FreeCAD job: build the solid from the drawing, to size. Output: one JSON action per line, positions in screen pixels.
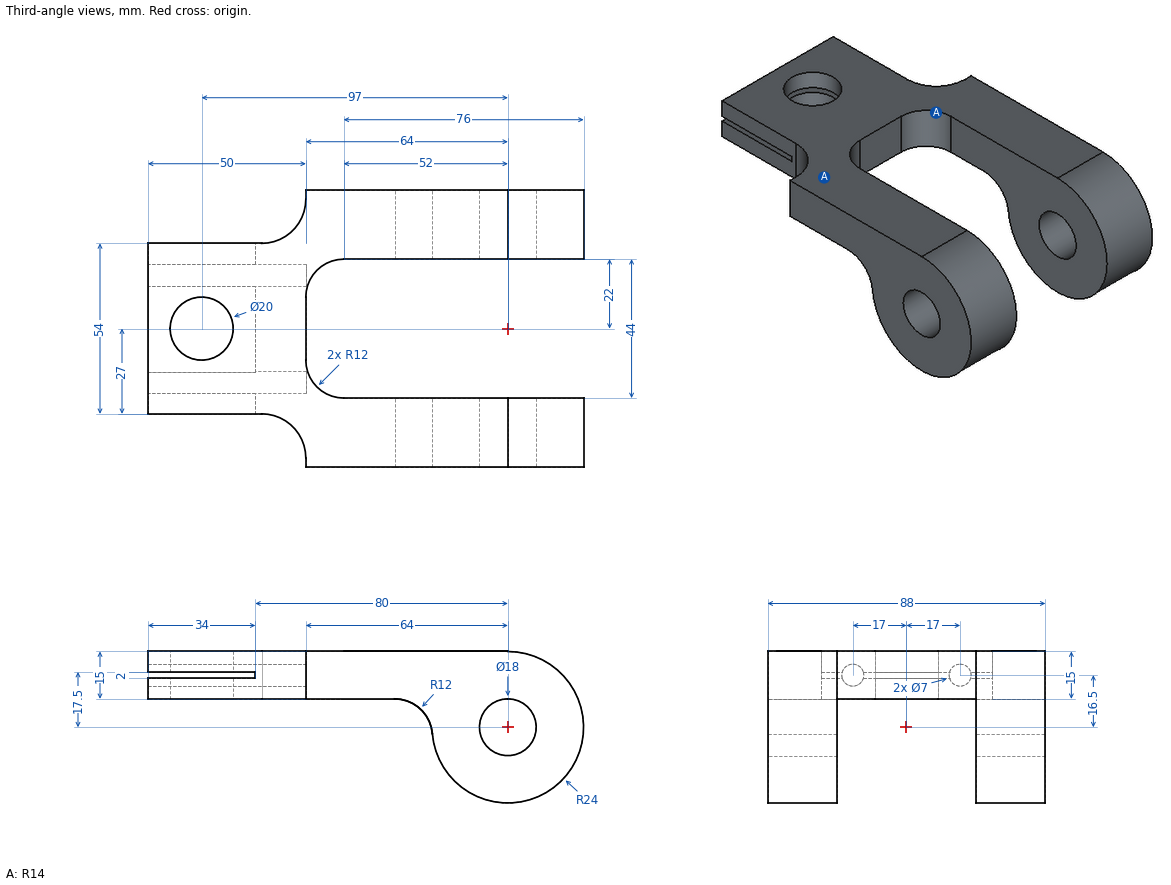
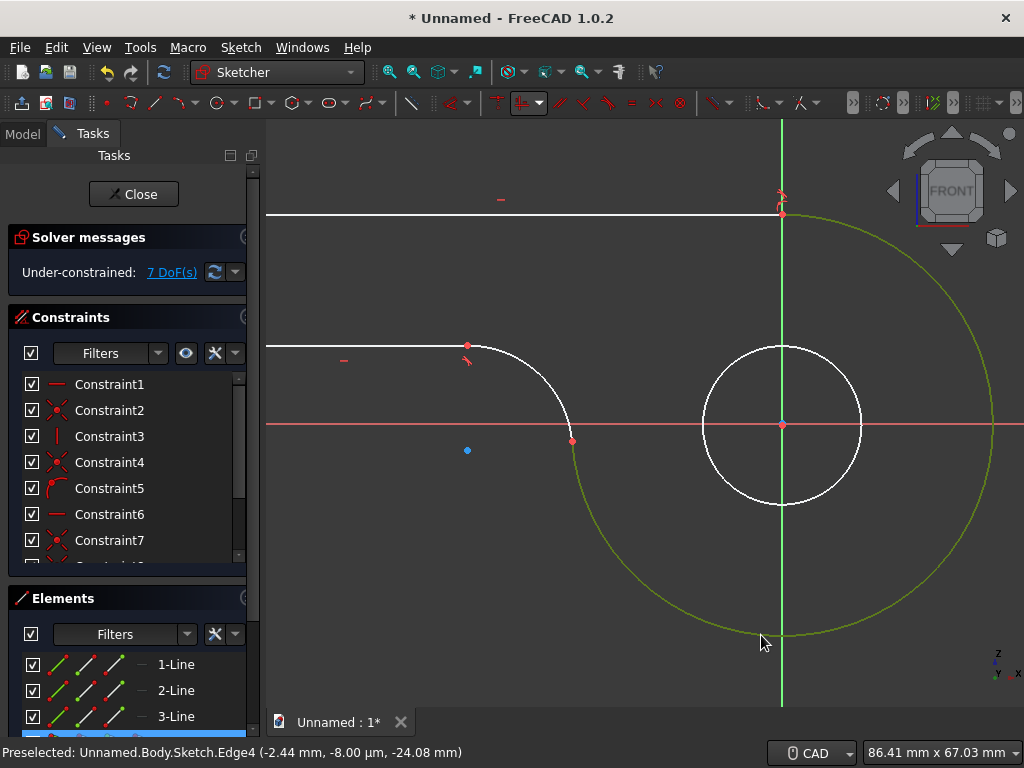
{"action": "left_click", "coordinate": [558, 398]}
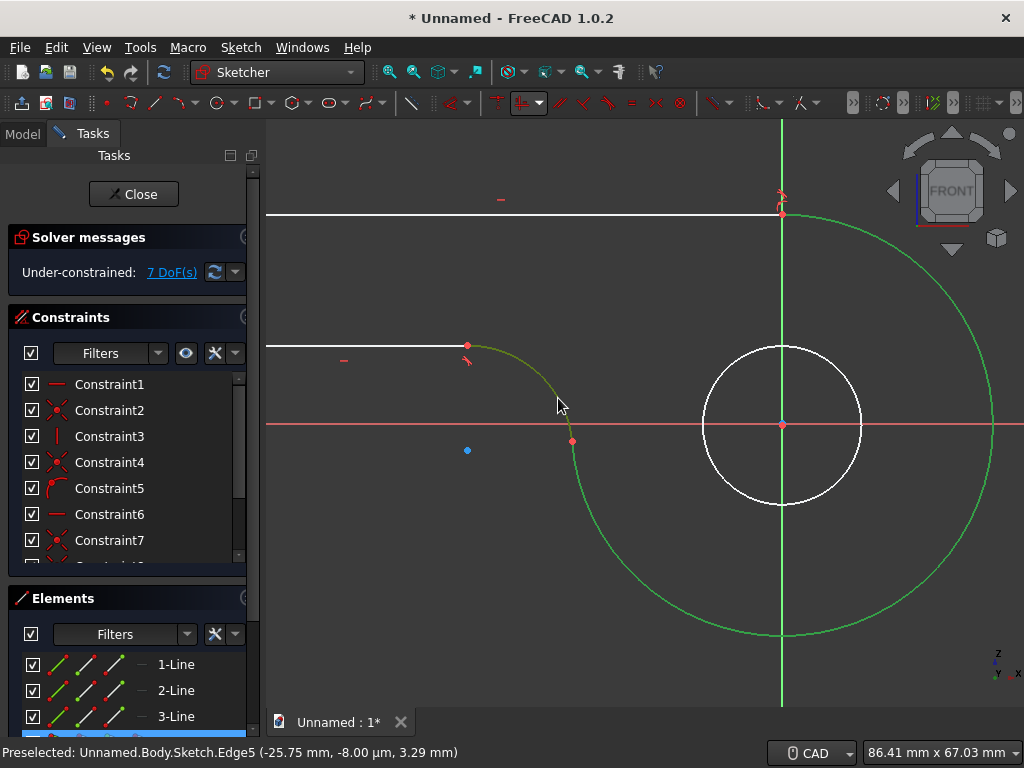
{"action": "left_click", "coordinate": [608, 104]}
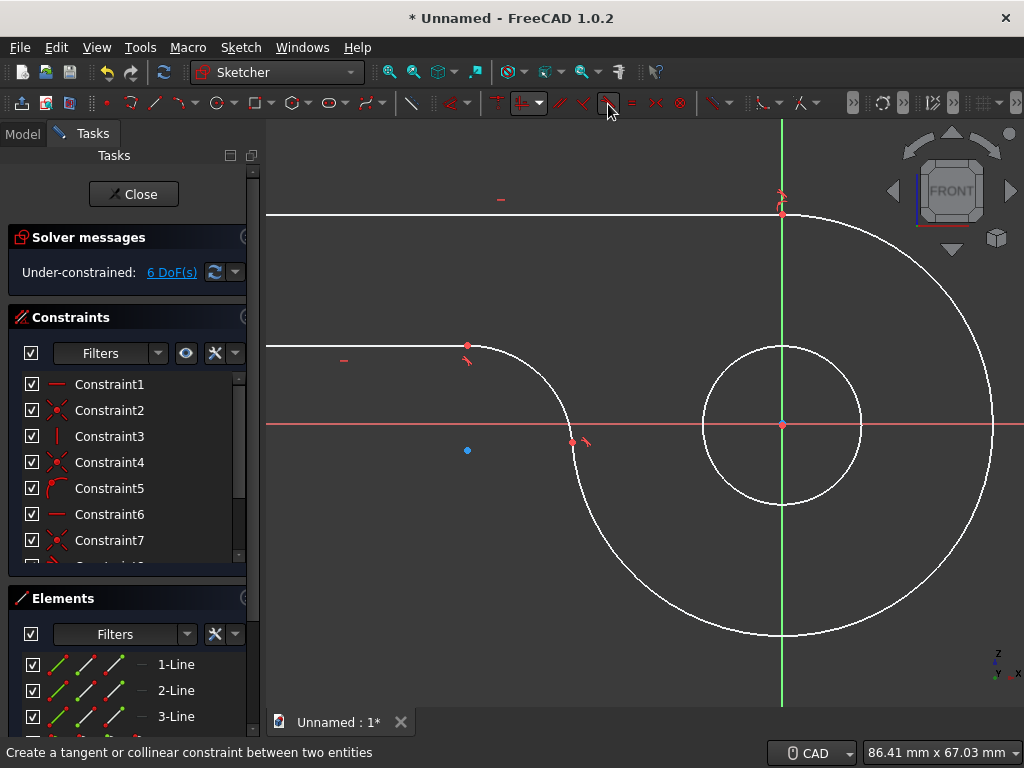
{"action": "left_click", "coordinate": [782, 425]}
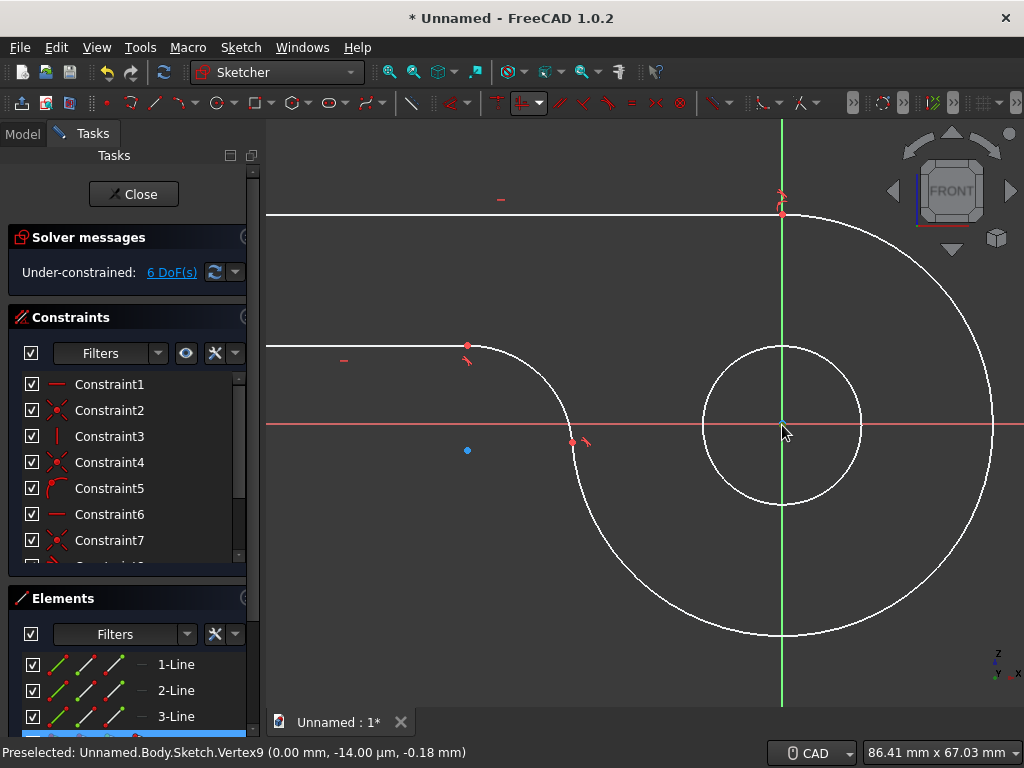
{"action": "left_click", "coordinate": [334, 424]}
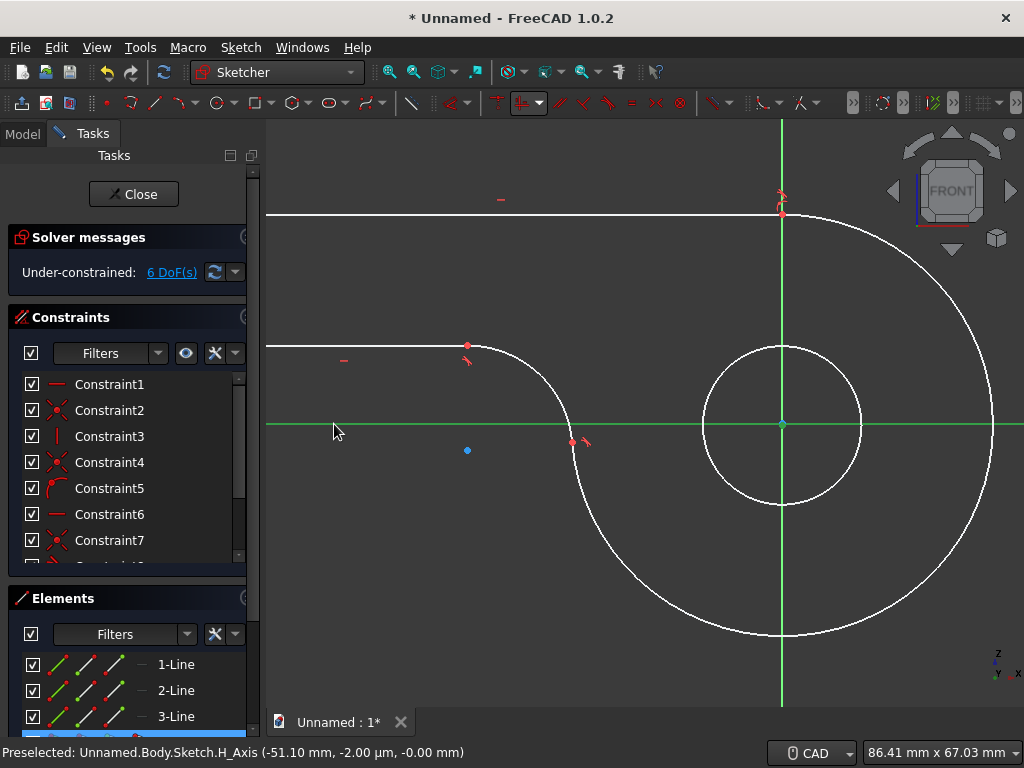
{"action": "left_click", "coordinate": [498, 104]}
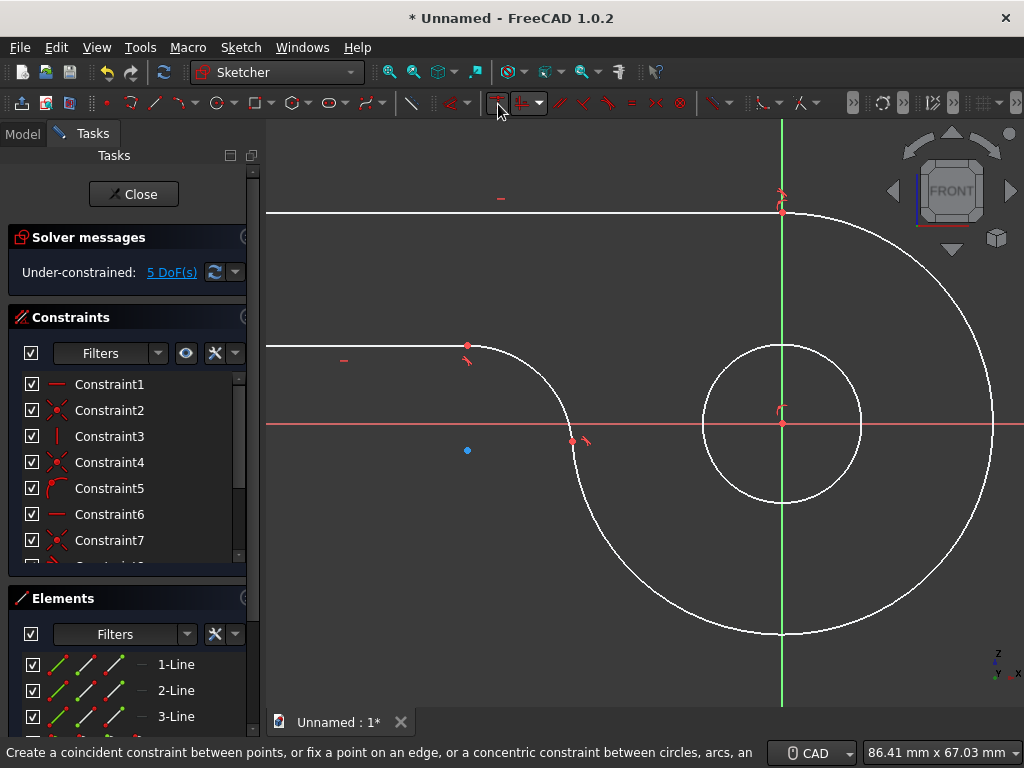
{"action": "left_click", "coordinate": [762, 634]}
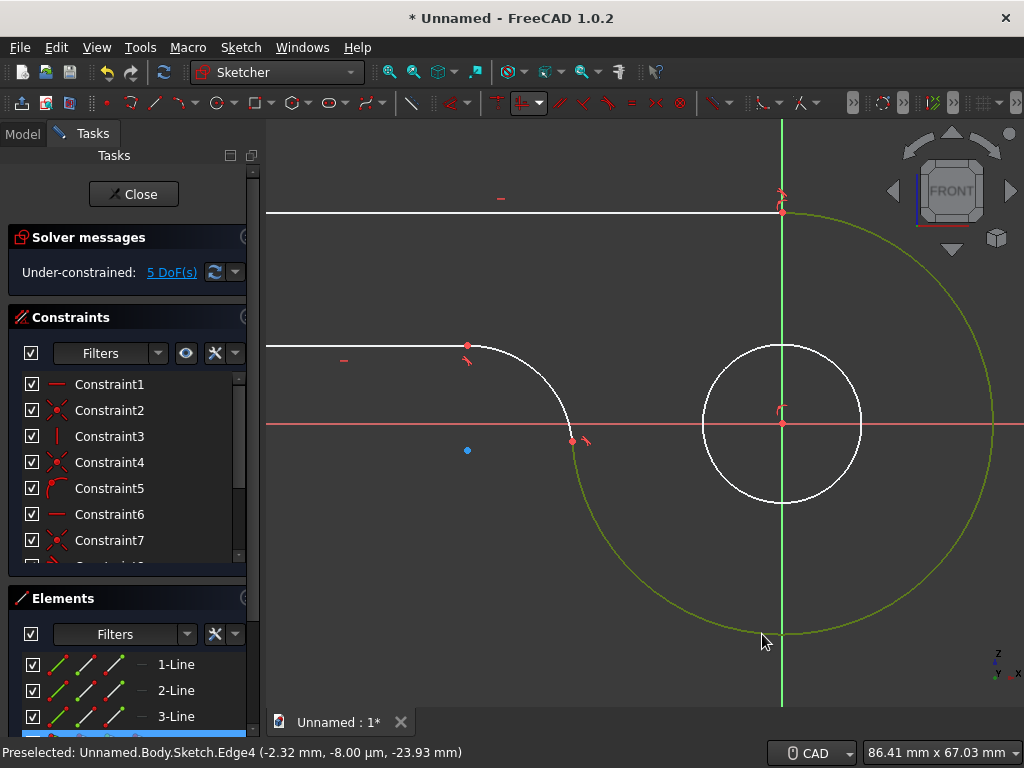
{"action": "key", "text": "k r"}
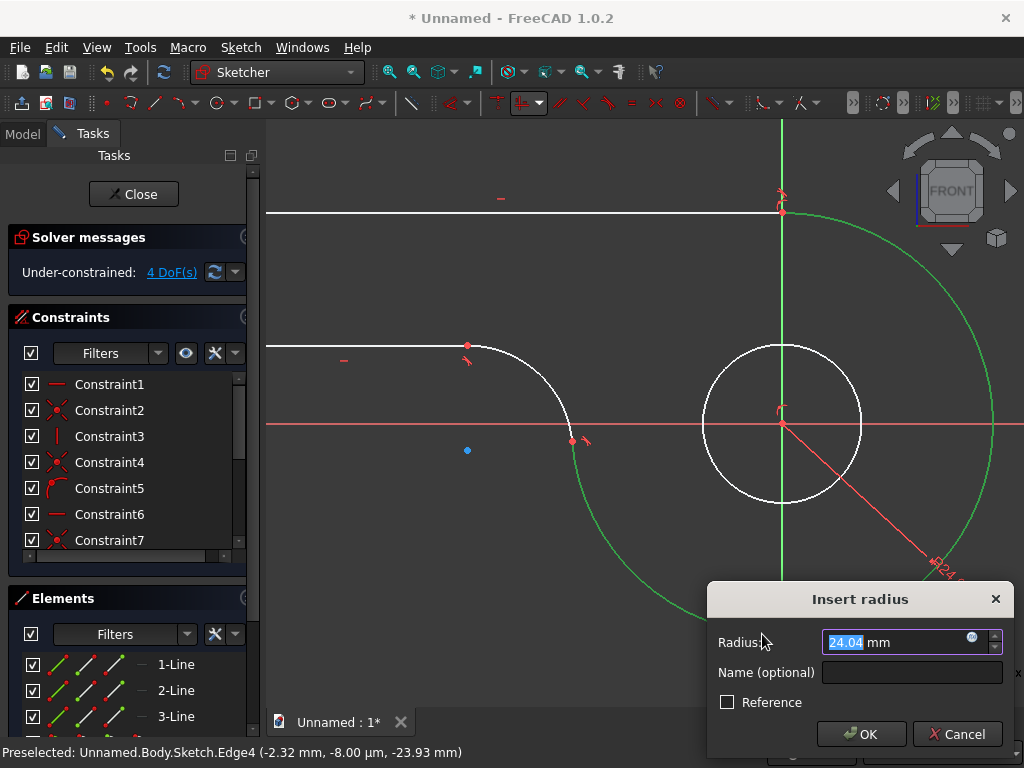
{"action": "type", "text": "24"}
{"action": "key", "text": "Return"}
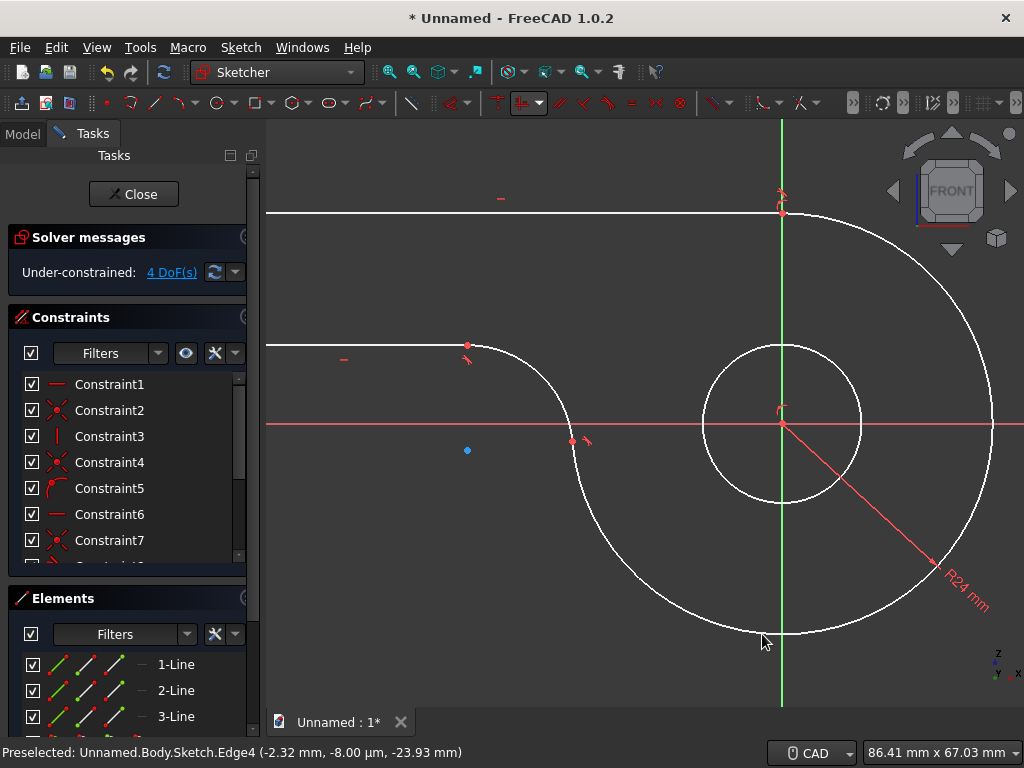
{"action": "left_click", "coordinate": [558, 397]}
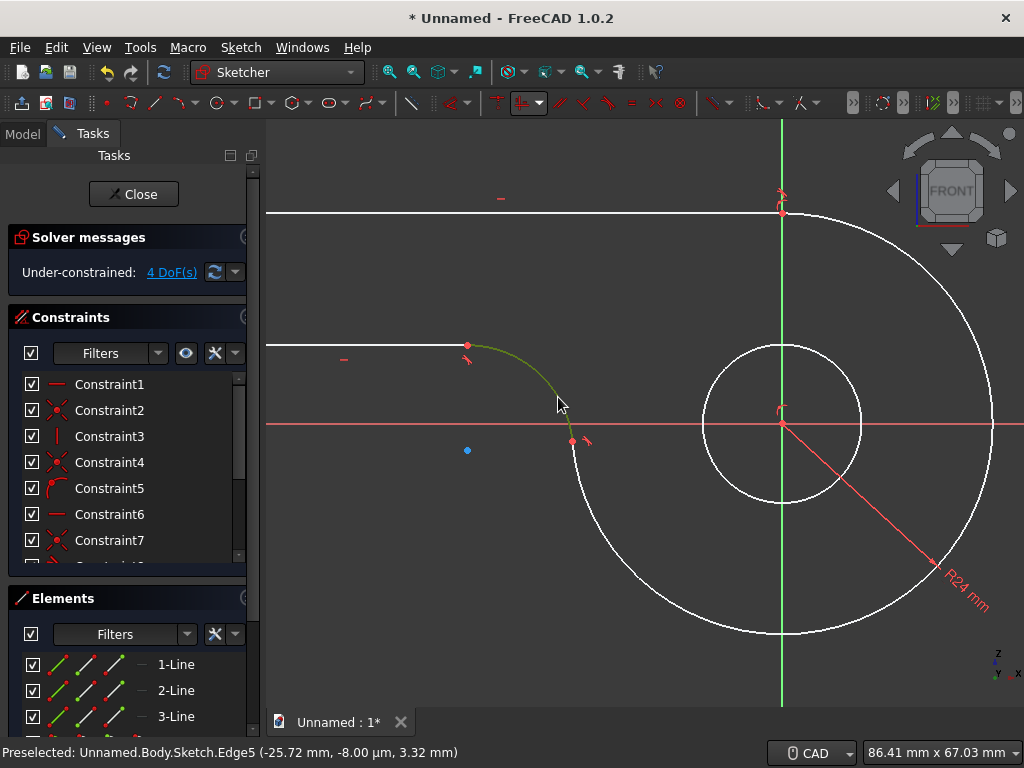
{"action": "left_click", "coordinate": [470, 104]}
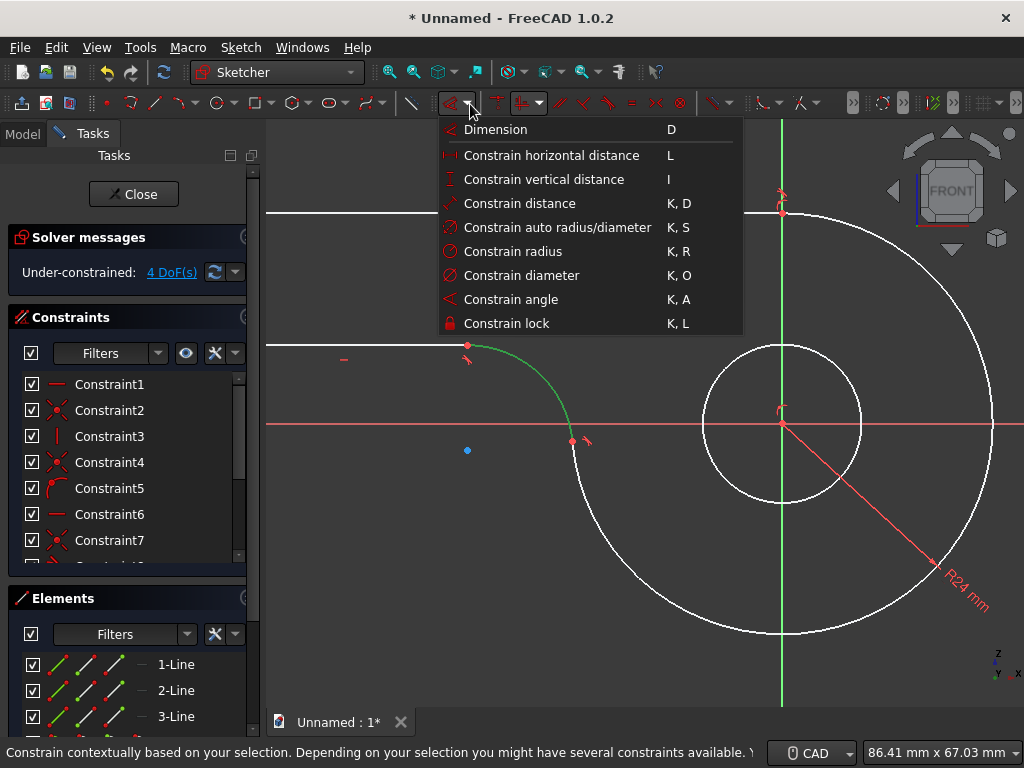
{"action": "left_click", "coordinate": [591, 251]}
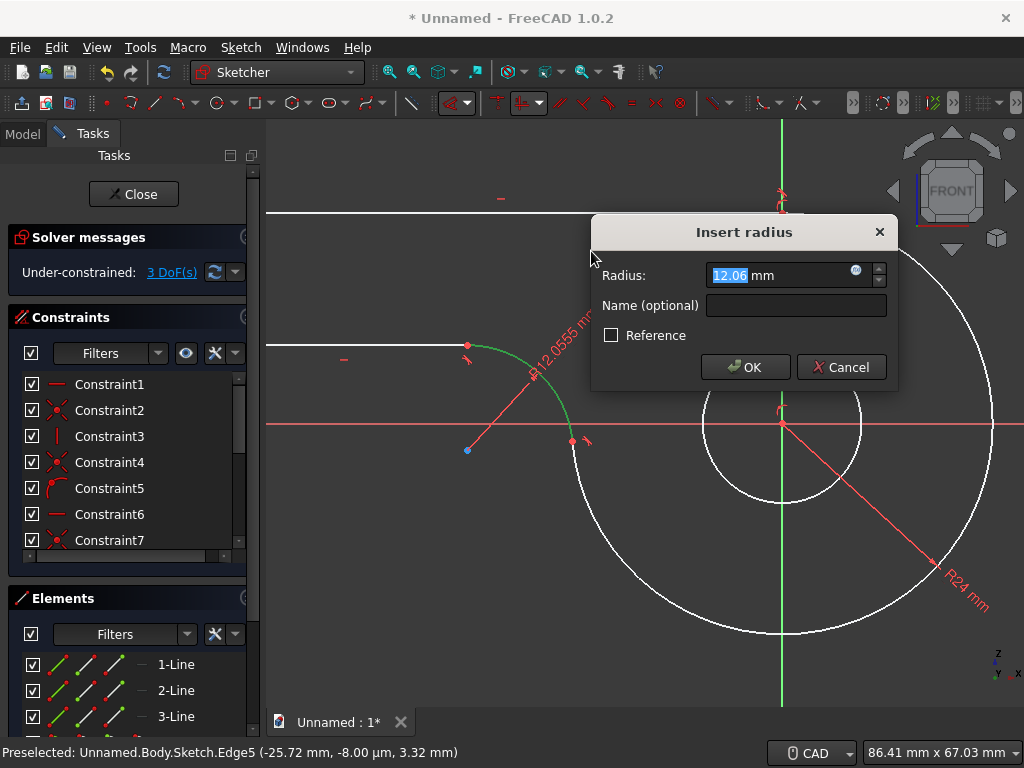
{"action": "type", "text": "12"}
{"action": "key", "text": "Return"}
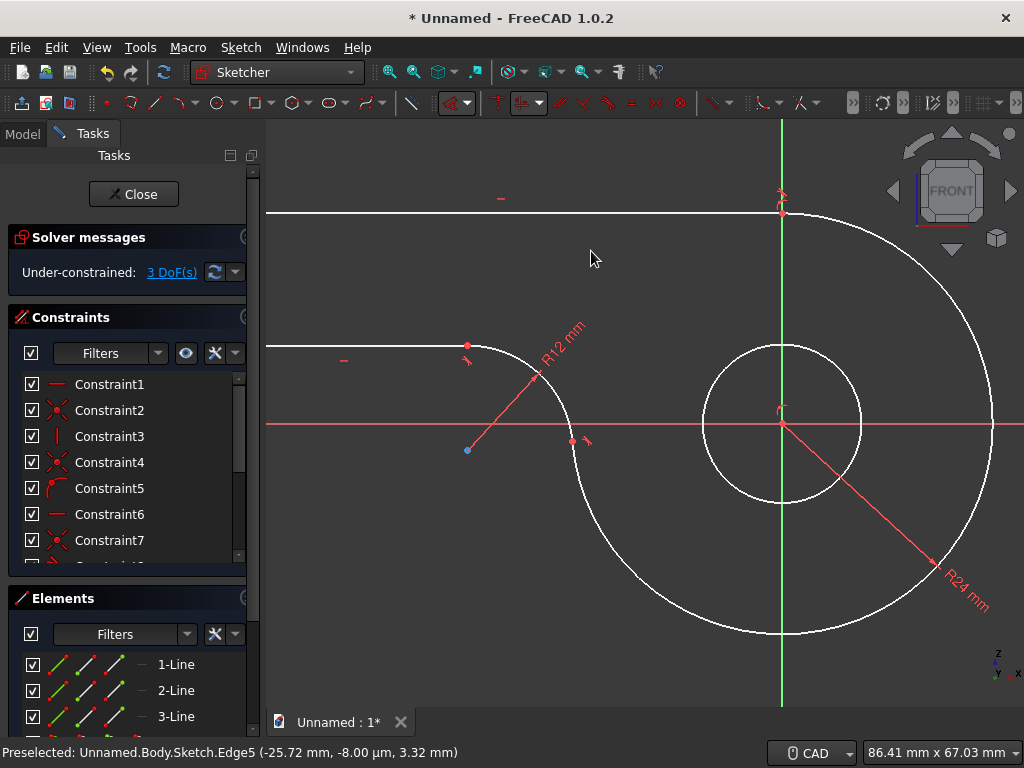
{"action": "left_click", "coordinate": [838, 368]}